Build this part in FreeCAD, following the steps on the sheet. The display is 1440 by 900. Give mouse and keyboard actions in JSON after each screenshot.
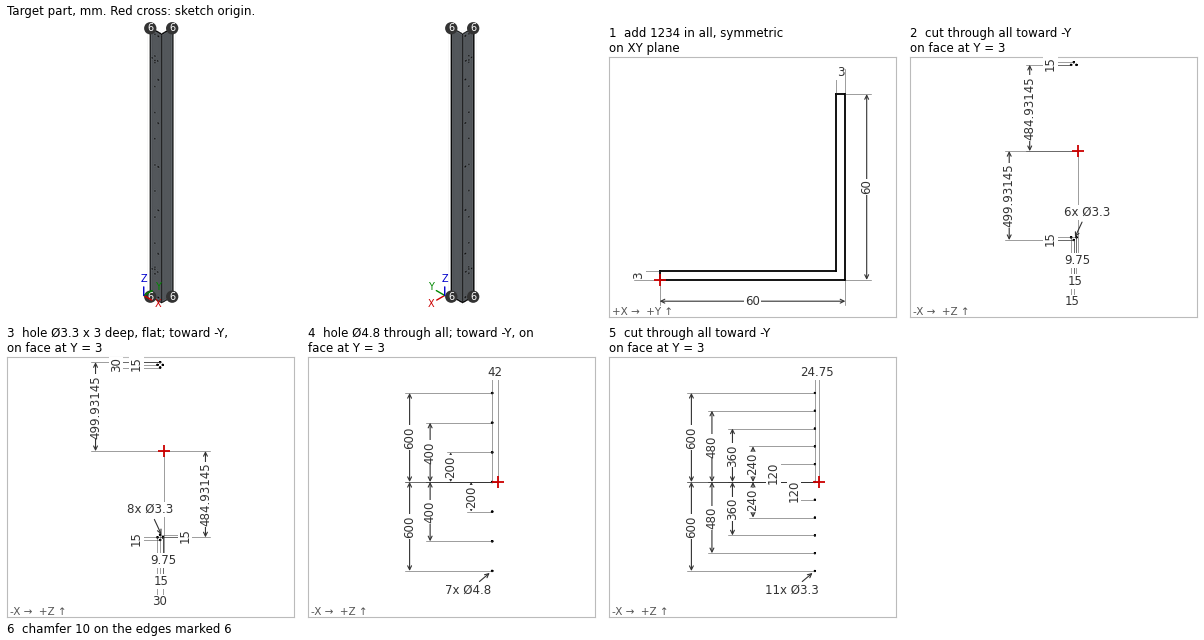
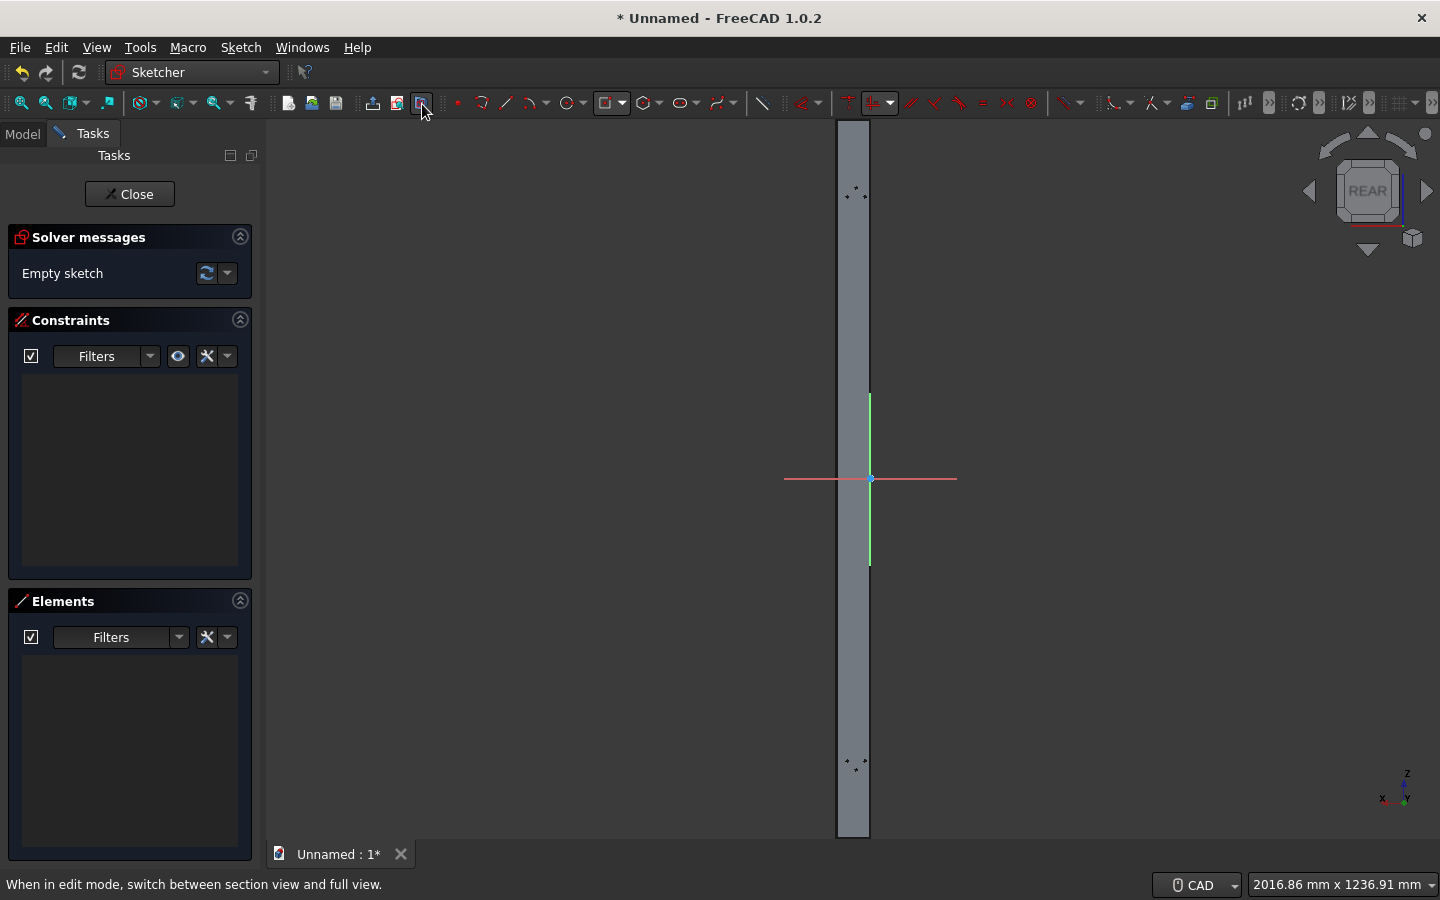
{"action": "left_click", "coordinate": [568, 104]}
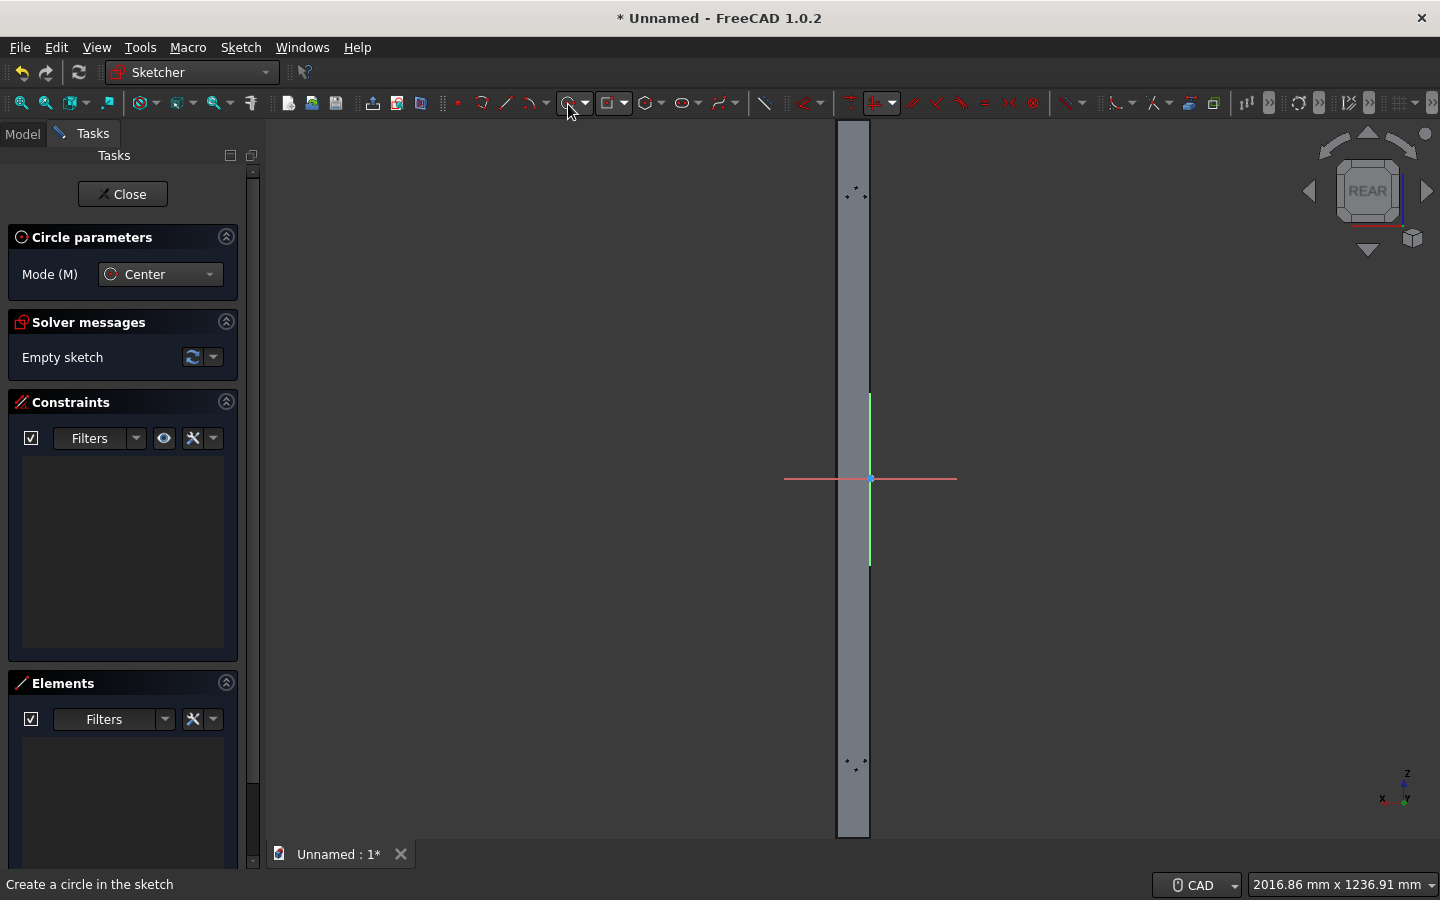
{"action": "scroll", "coordinate": [865, 761], "scroll_direction": "up", "scroll_amount": 16}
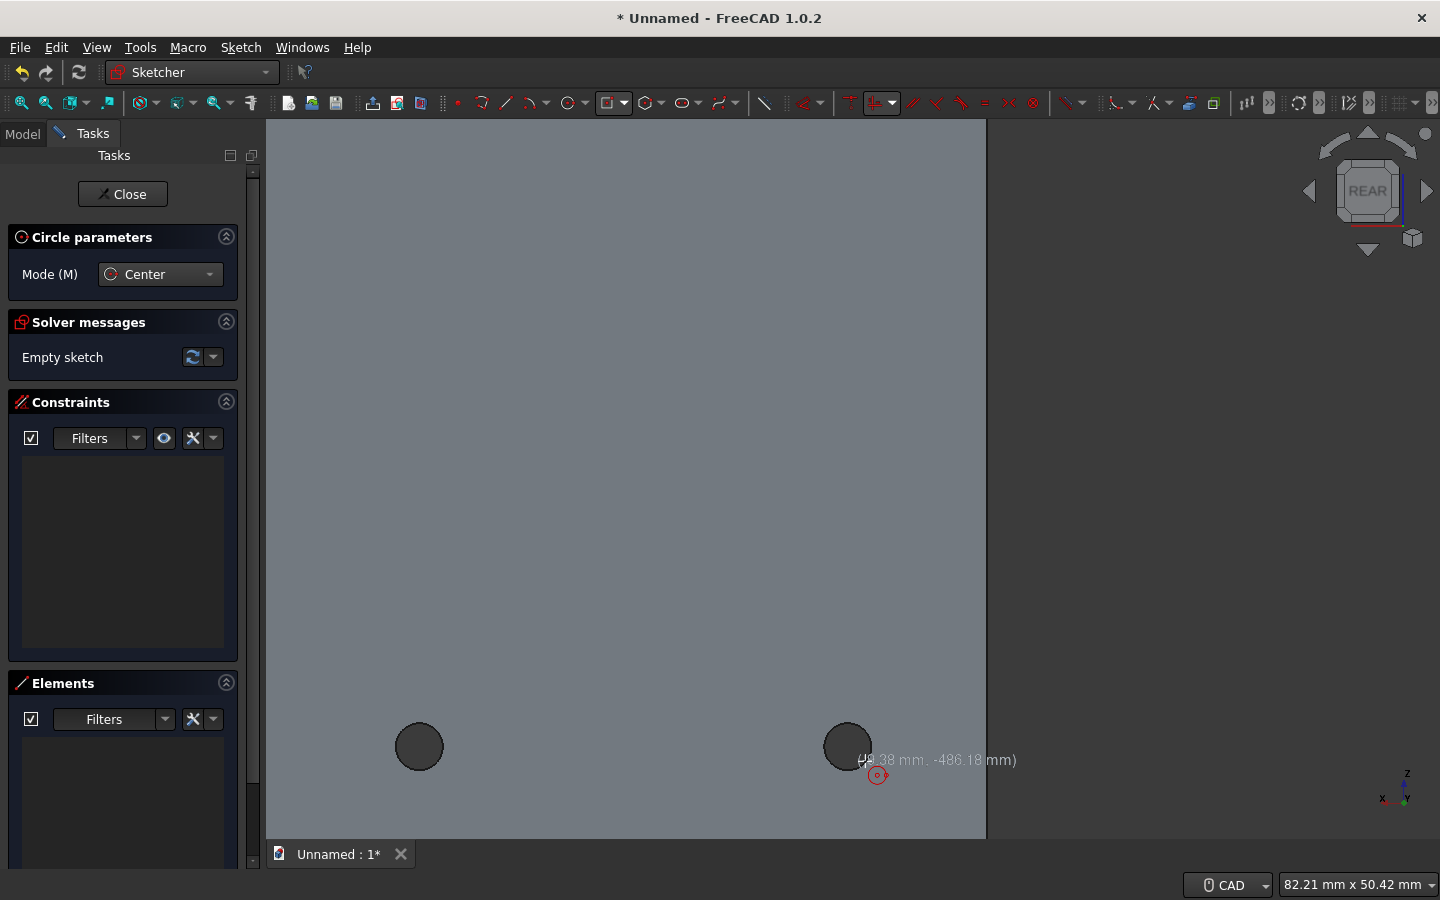
{"action": "scroll", "coordinate": [788, 762], "scroll_direction": "down", "scroll_amount": 16}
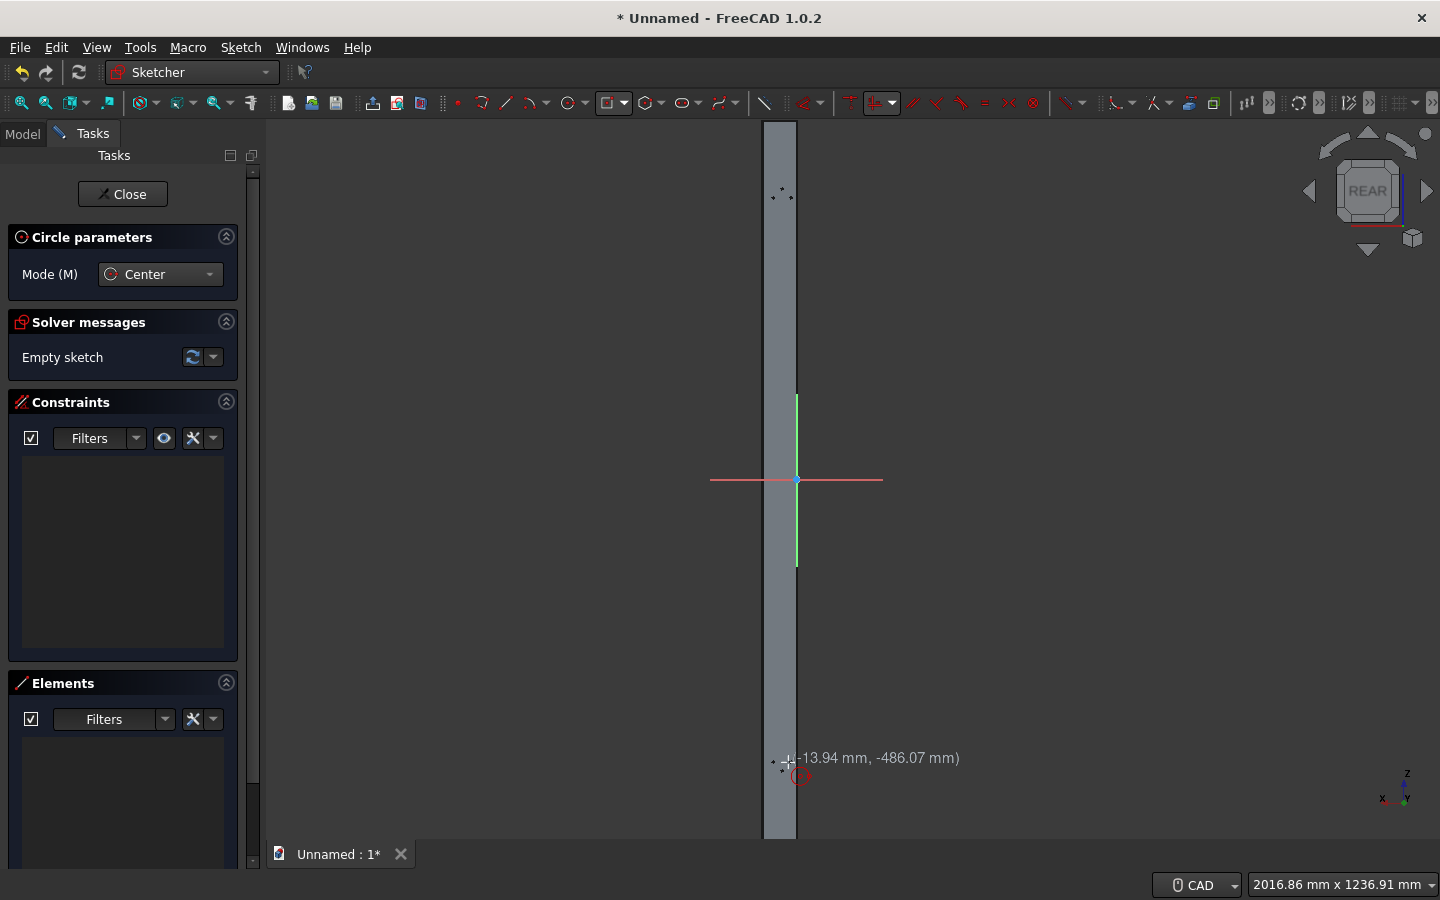
{"action": "scroll", "coordinate": [791, 762], "scroll_direction": "up", "scroll_amount": 6}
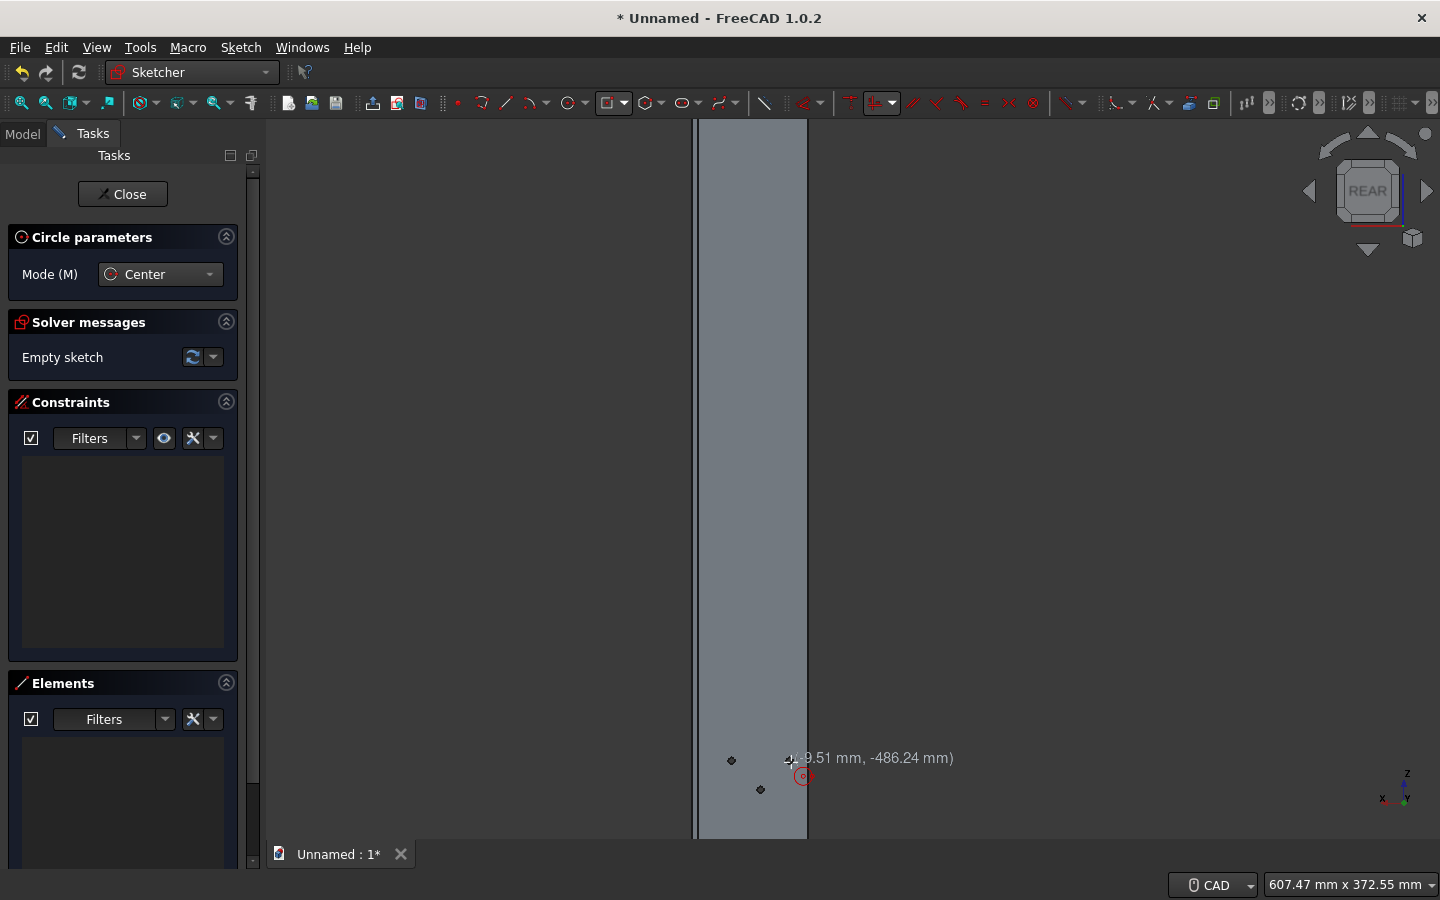
{"action": "left_click", "coordinate": [790, 761]}
{"action": "mouse_move", "coordinate": [792, 758]}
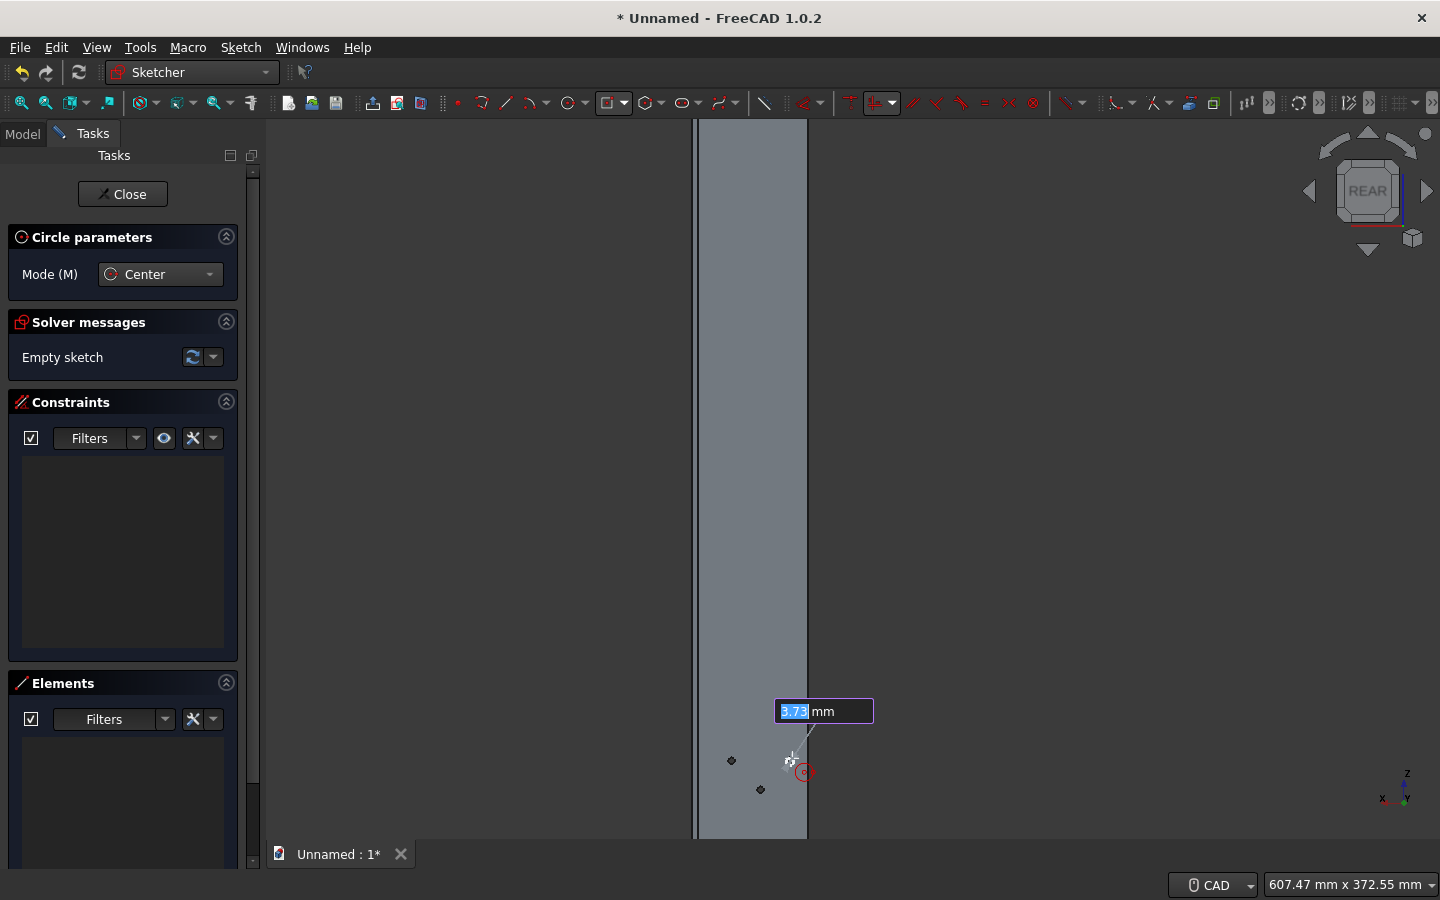
{"action": "type", "text": "3.3"}
{"action": "key", "text": "Return"}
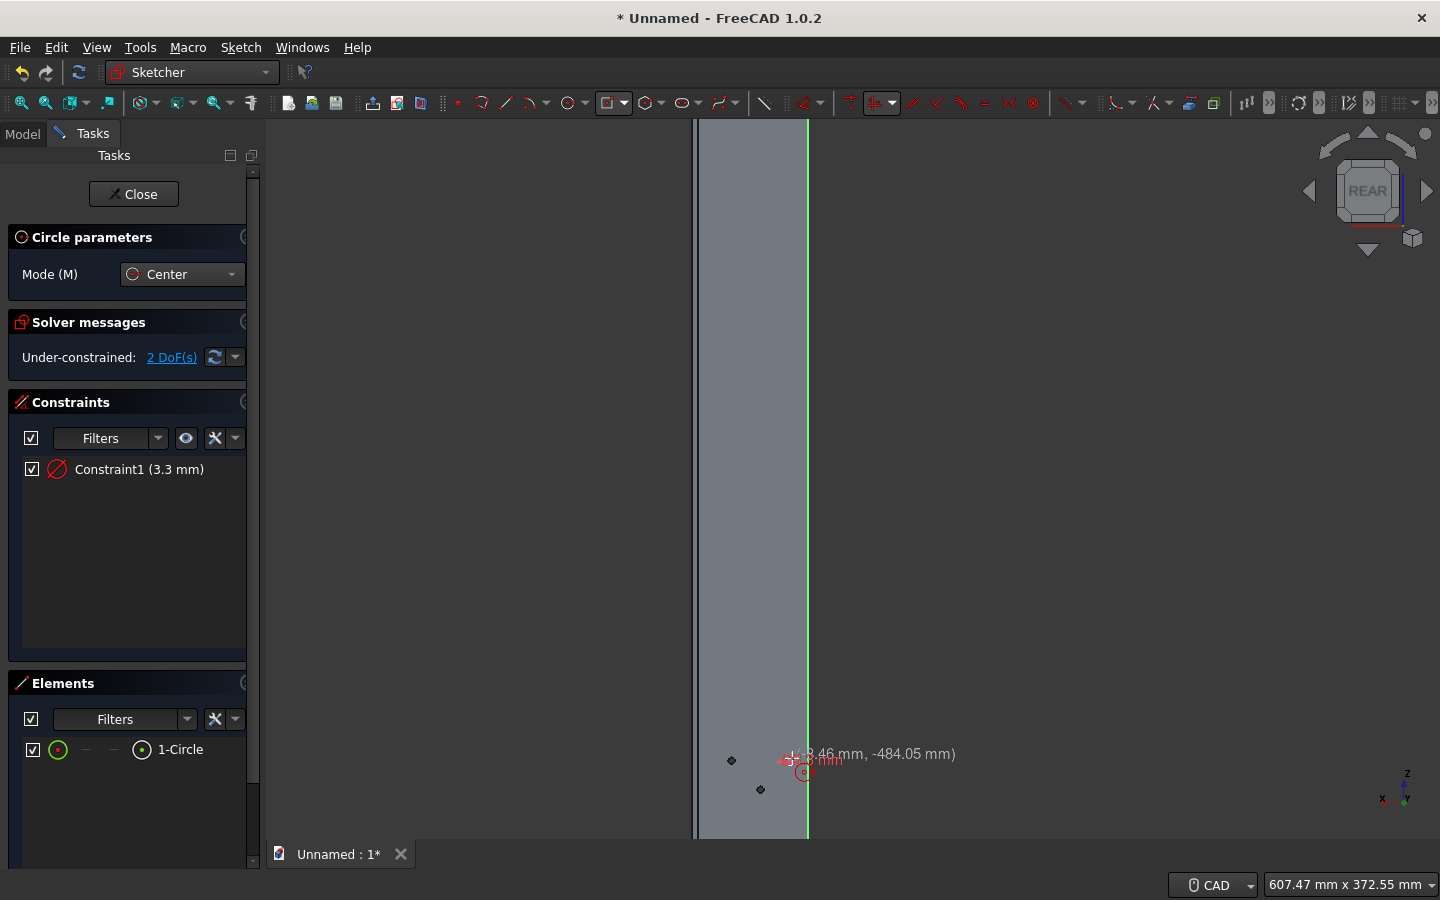
{"action": "scroll", "coordinate": [732, 761], "scroll_direction": "up", "scroll_amount": 10}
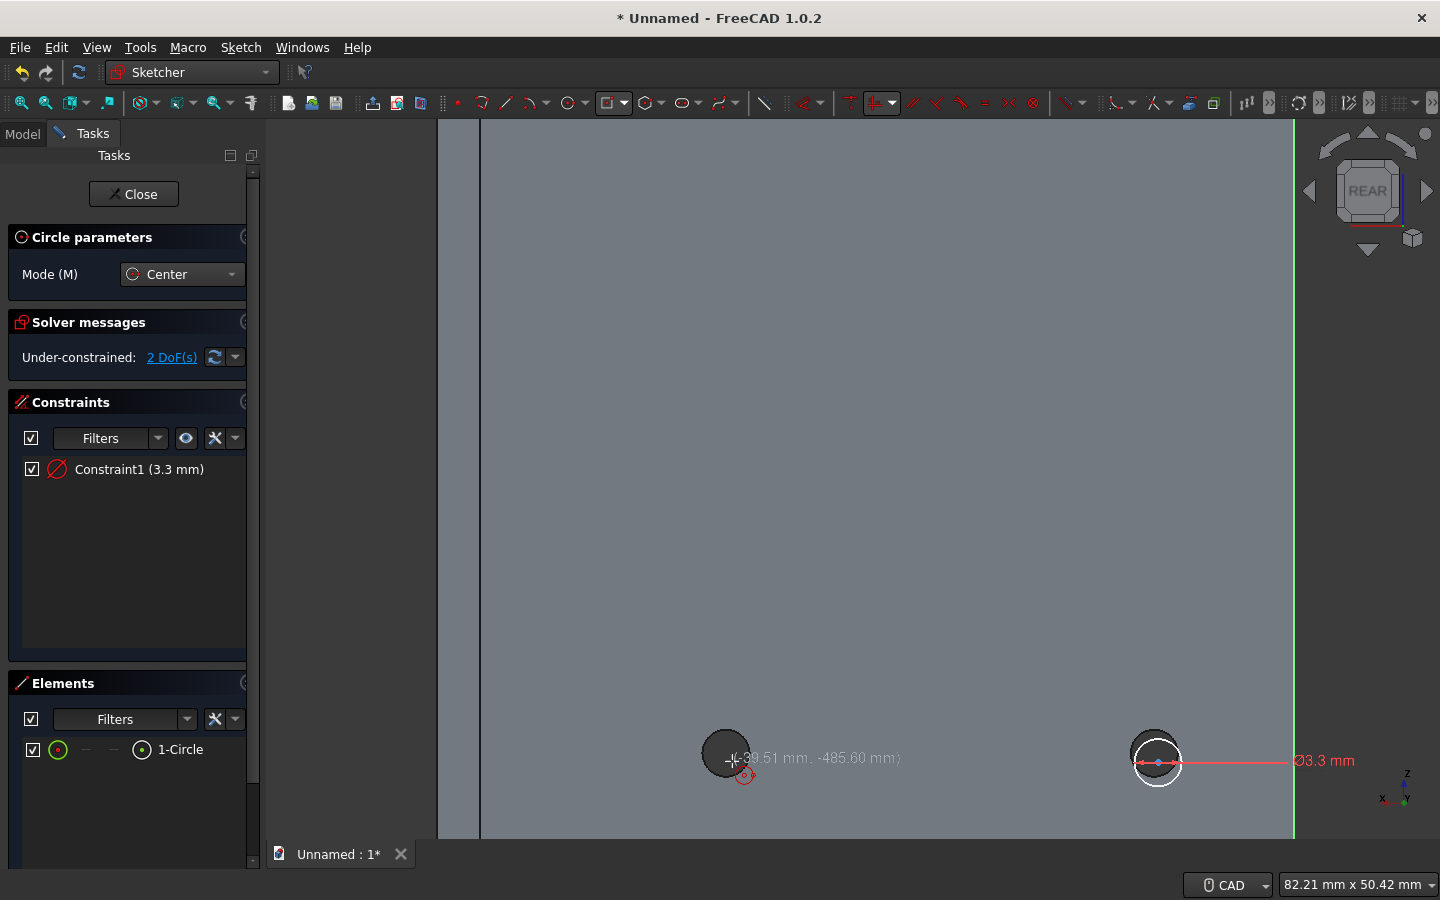
{"action": "scroll", "coordinate": [775, 762], "scroll_direction": "down", "scroll_amount": 16}